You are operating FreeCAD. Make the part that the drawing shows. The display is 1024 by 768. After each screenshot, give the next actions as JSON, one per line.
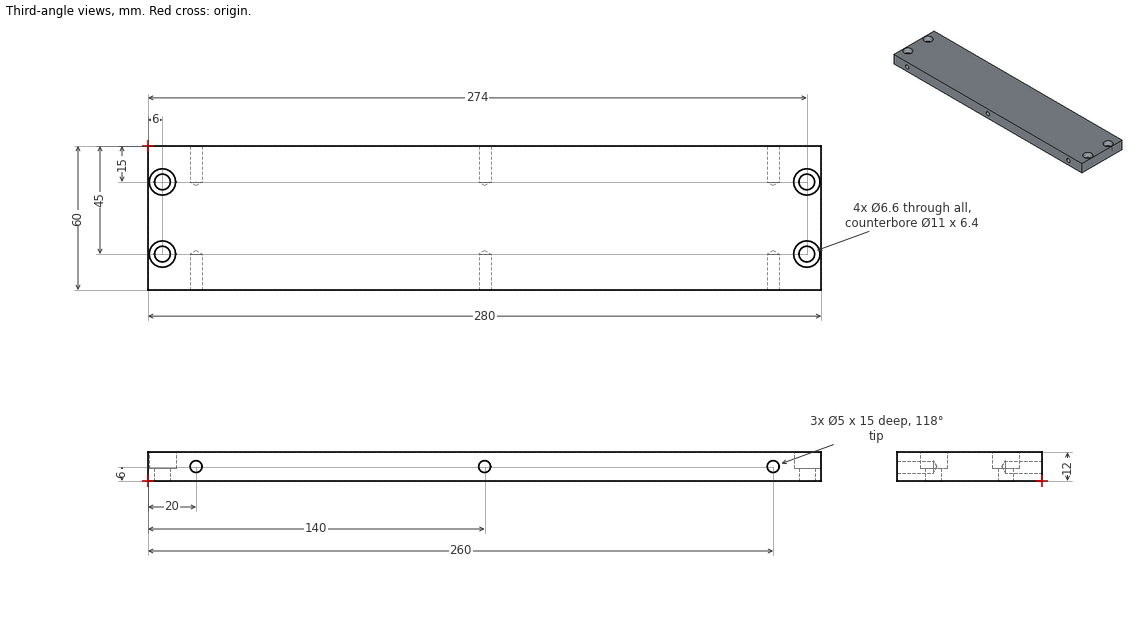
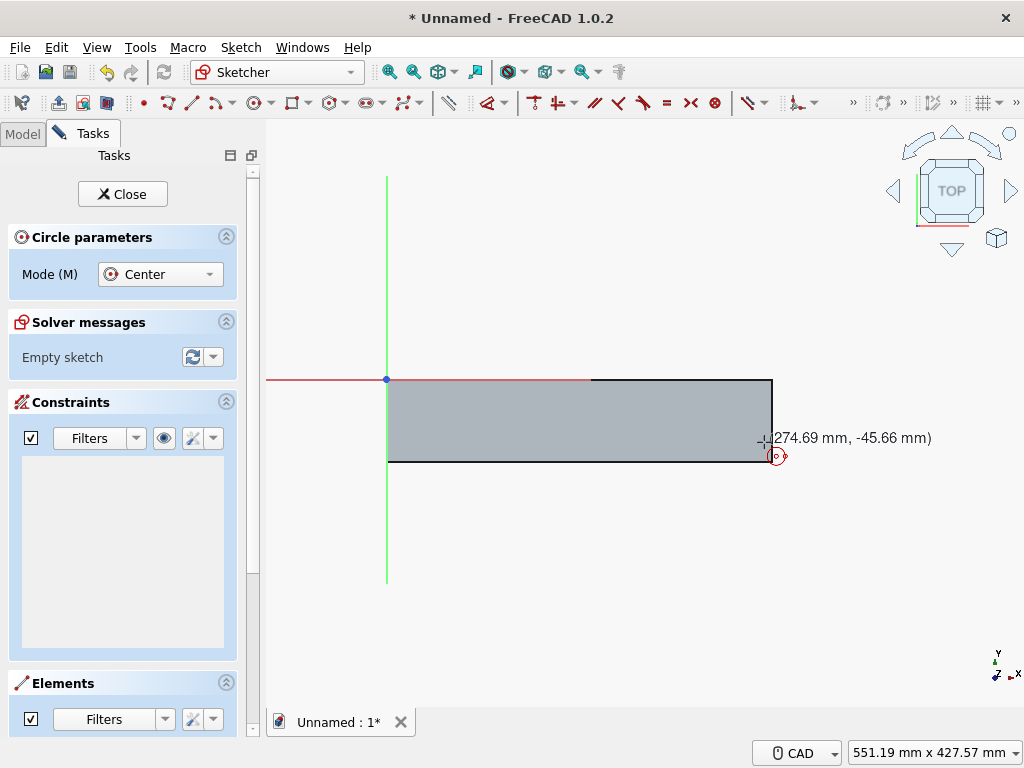
{"action": "left_click", "coordinate": [764, 442]}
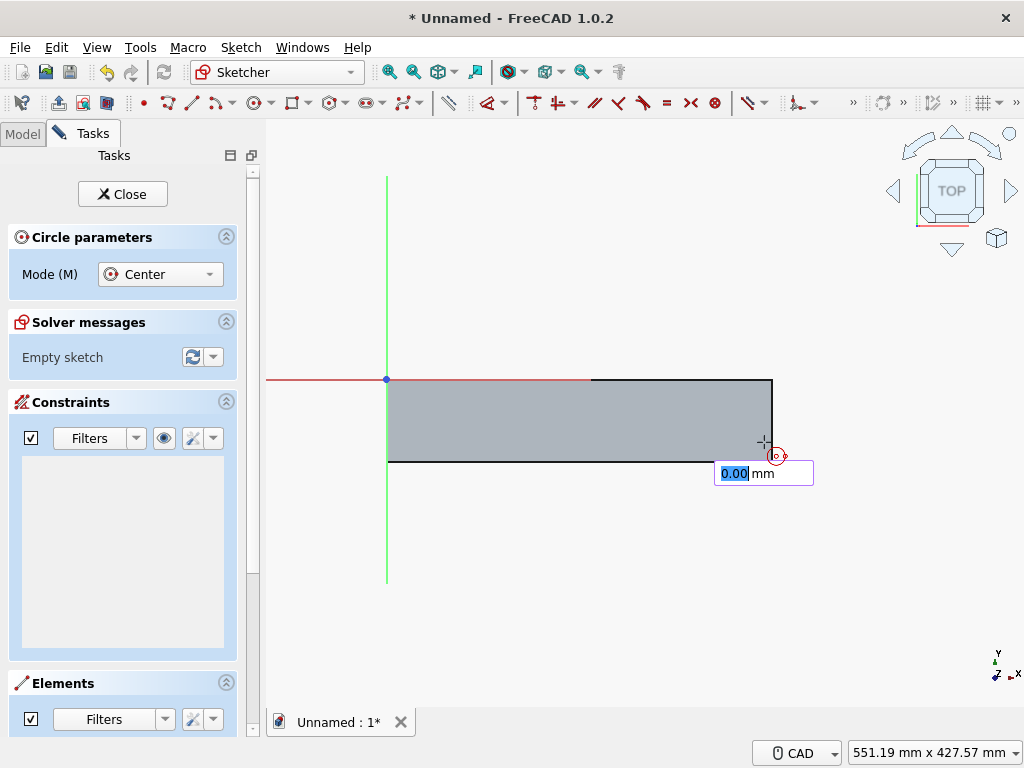
{"action": "scroll", "coordinate": [767, 439], "scroll_direction": "up", "scroll_amount": 7}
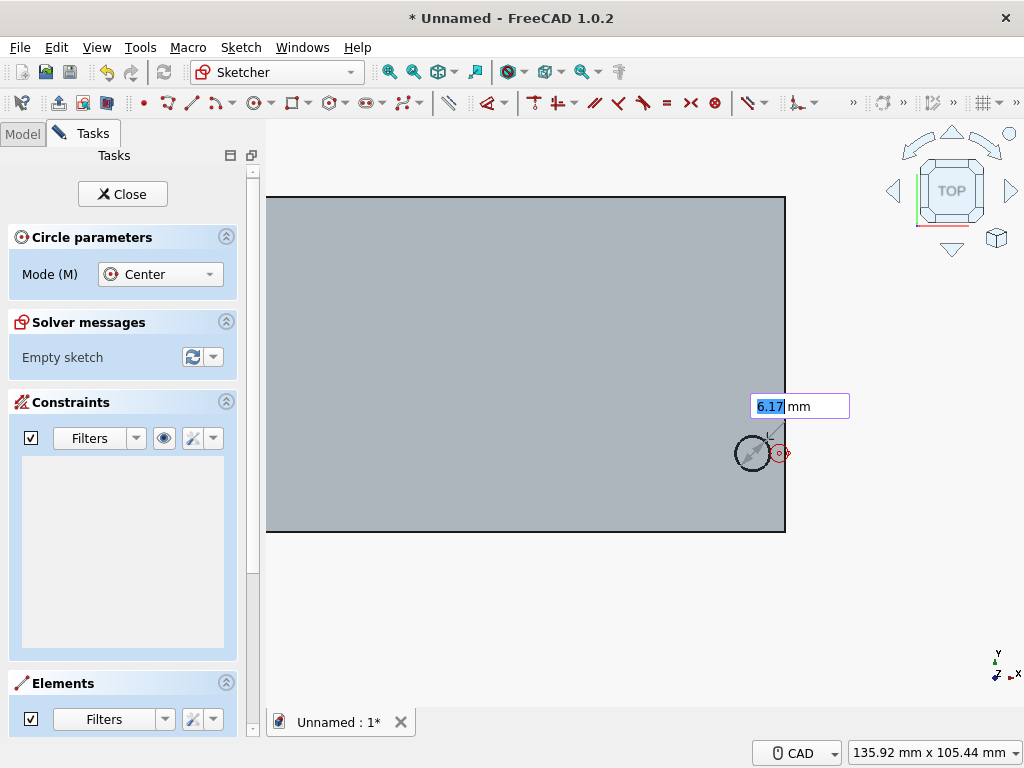
{"action": "left_click", "coordinate": [764, 435]}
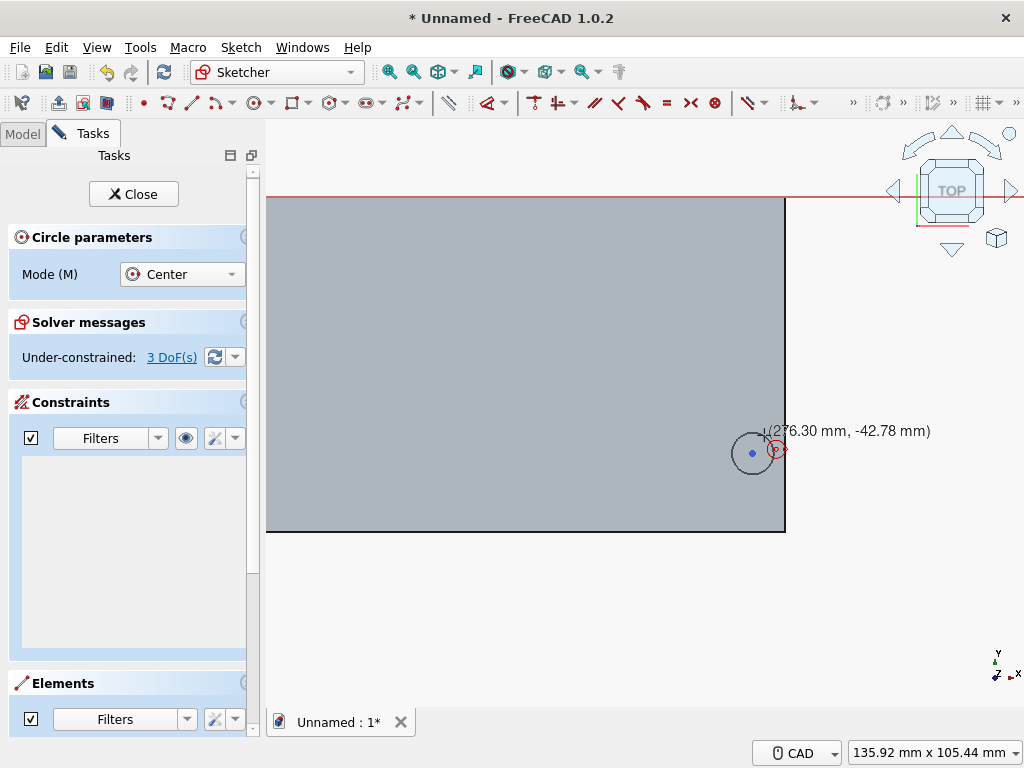
{"action": "scroll", "coordinate": [751, 281], "scroll_direction": "up", "scroll_amount": 2}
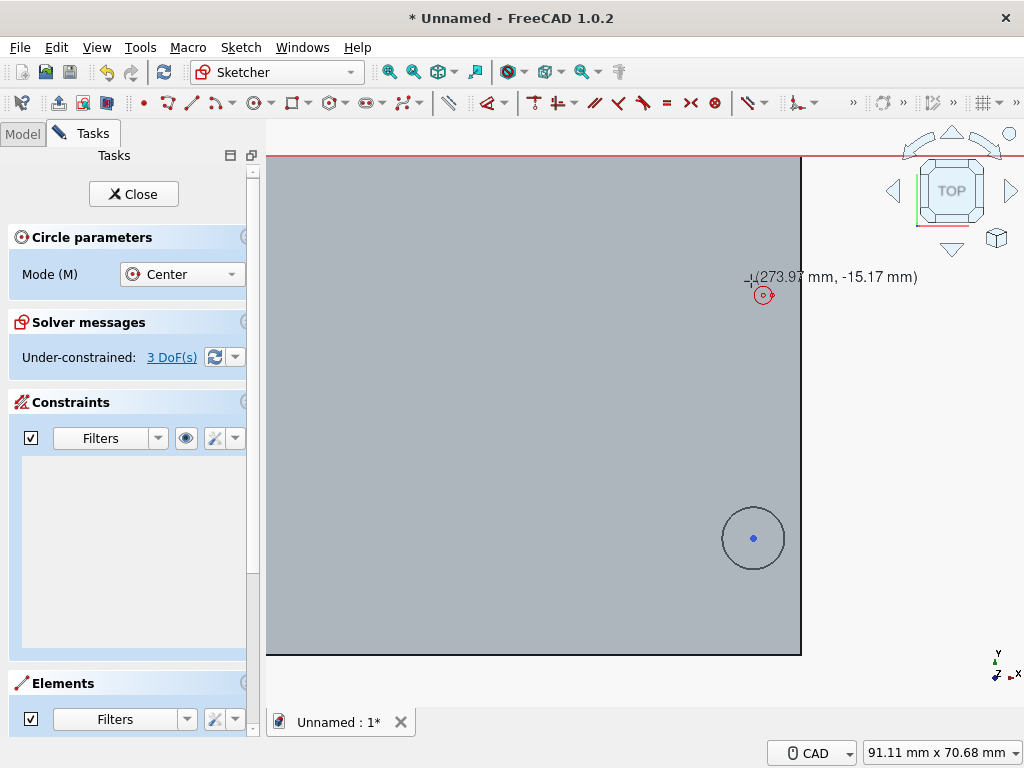
{"action": "scroll", "coordinate": [765, 424], "scroll_direction": "down", "scroll_amount": 9}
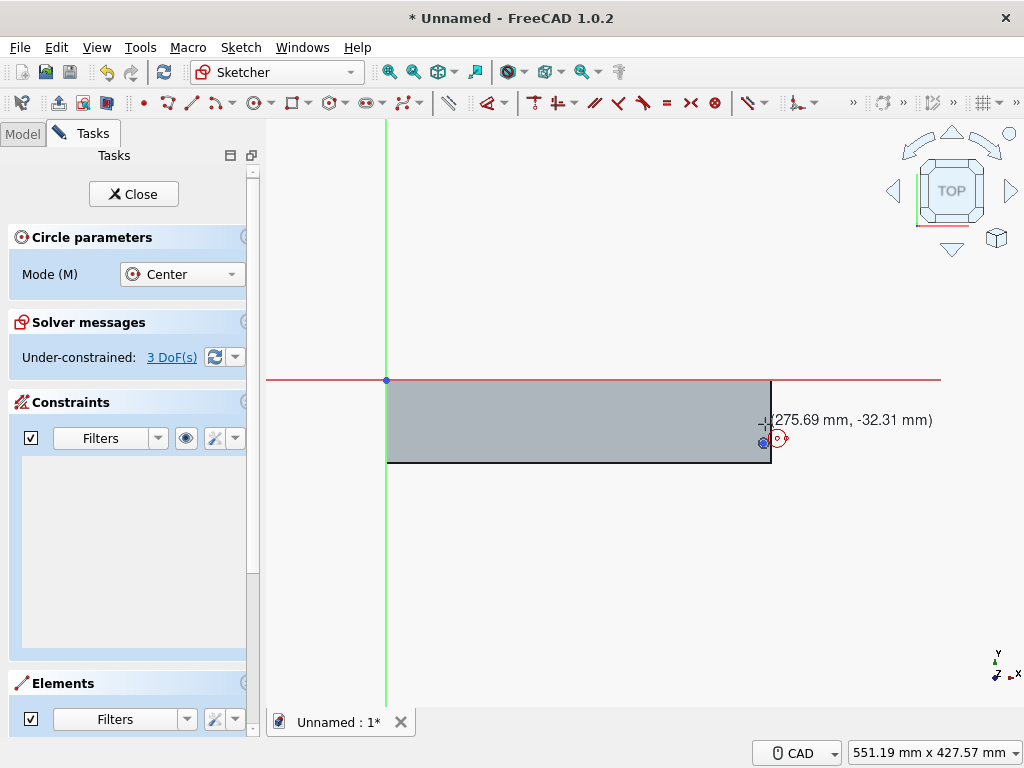
{"action": "left_click", "coordinate": [763, 401]}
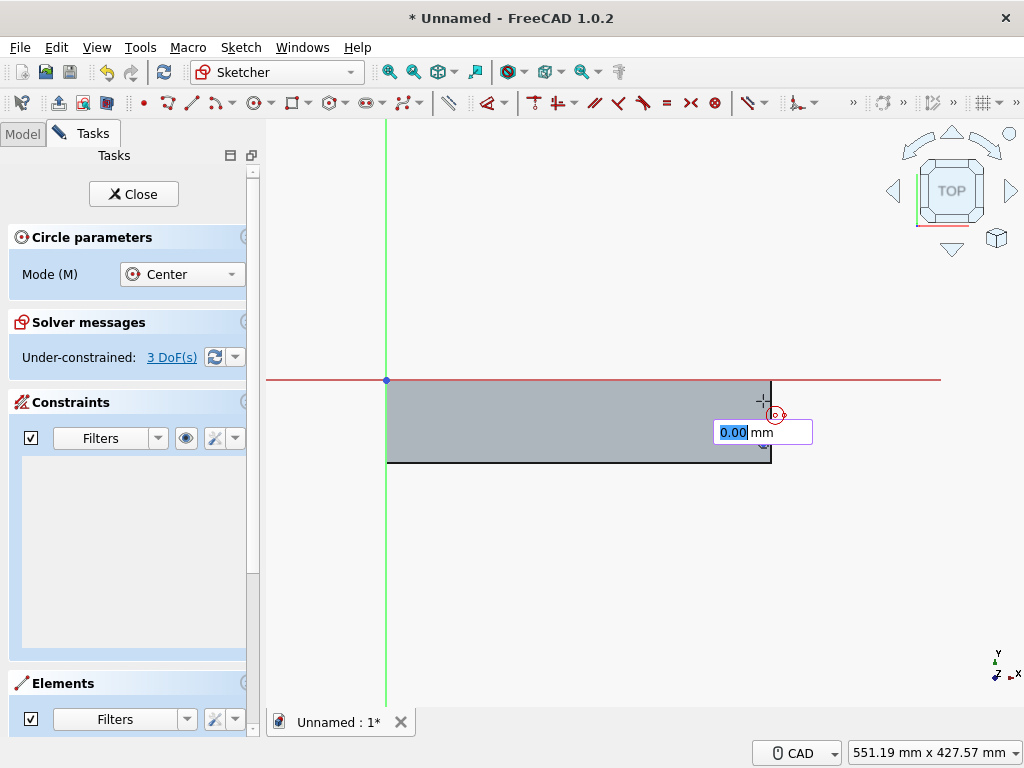
{"action": "scroll", "coordinate": [766, 398], "scroll_direction": "up", "scroll_amount": 7}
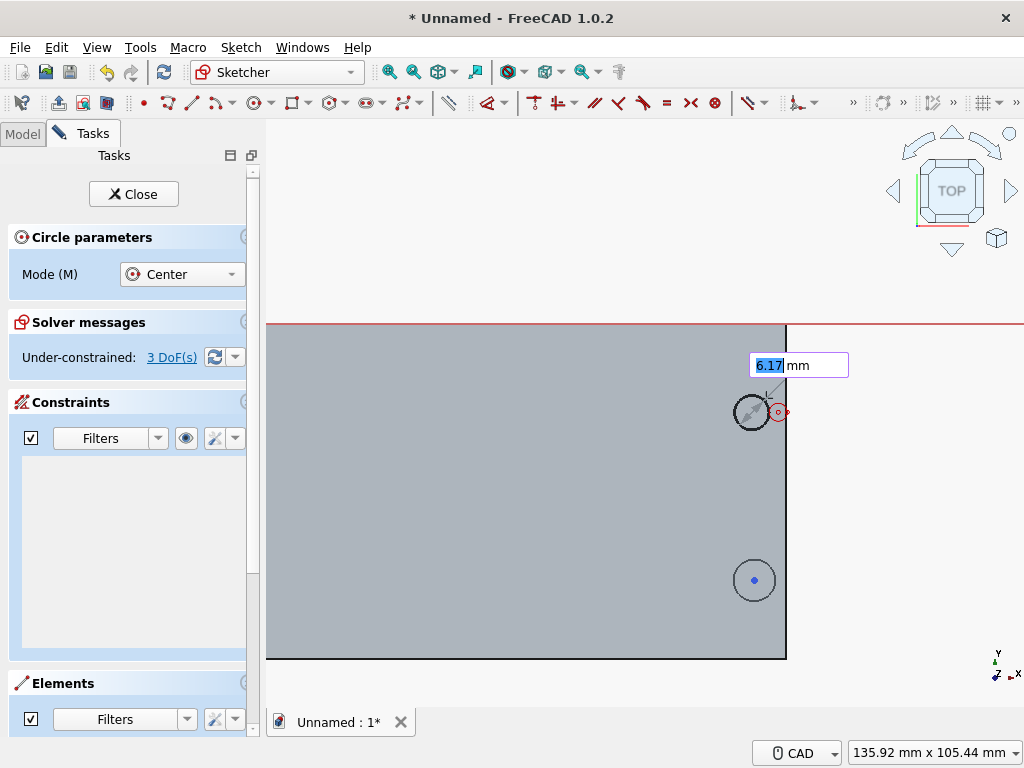
{"action": "left_click", "coordinate": [766, 395]}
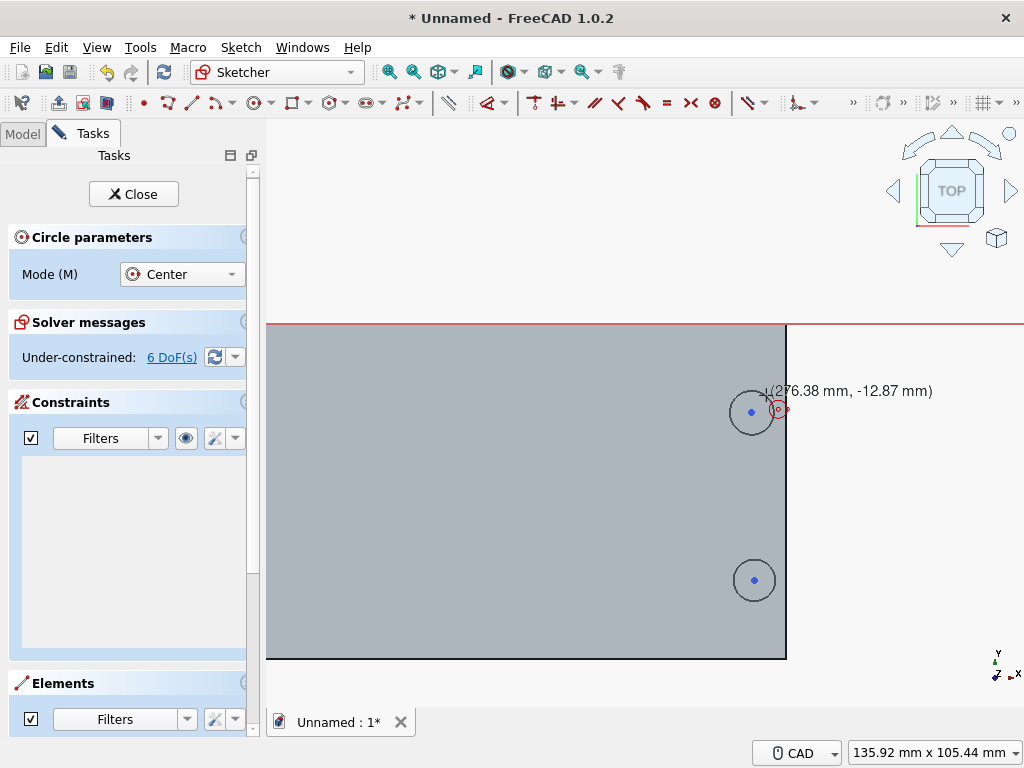
{"action": "scroll", "coordinate": [766, 398], "scroll_direction": "down", "scroll_amount": 7}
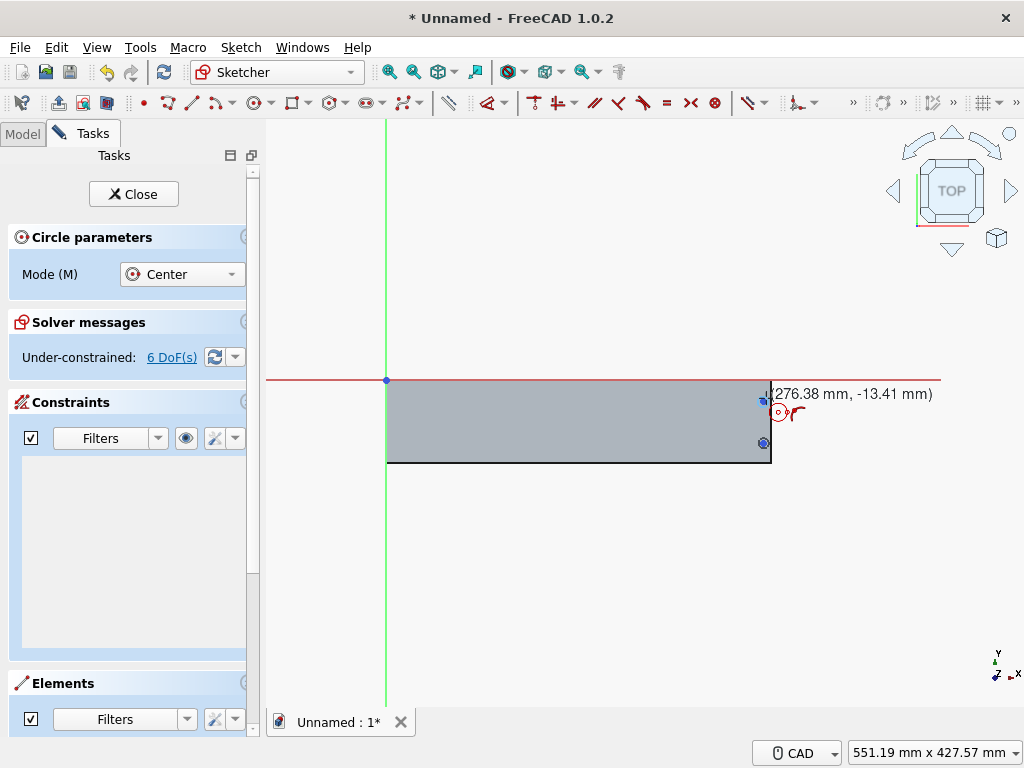
{"action": "scroll", "coordinate": [395, 442], "scroll_direction": "up", "scroll_amount": 9}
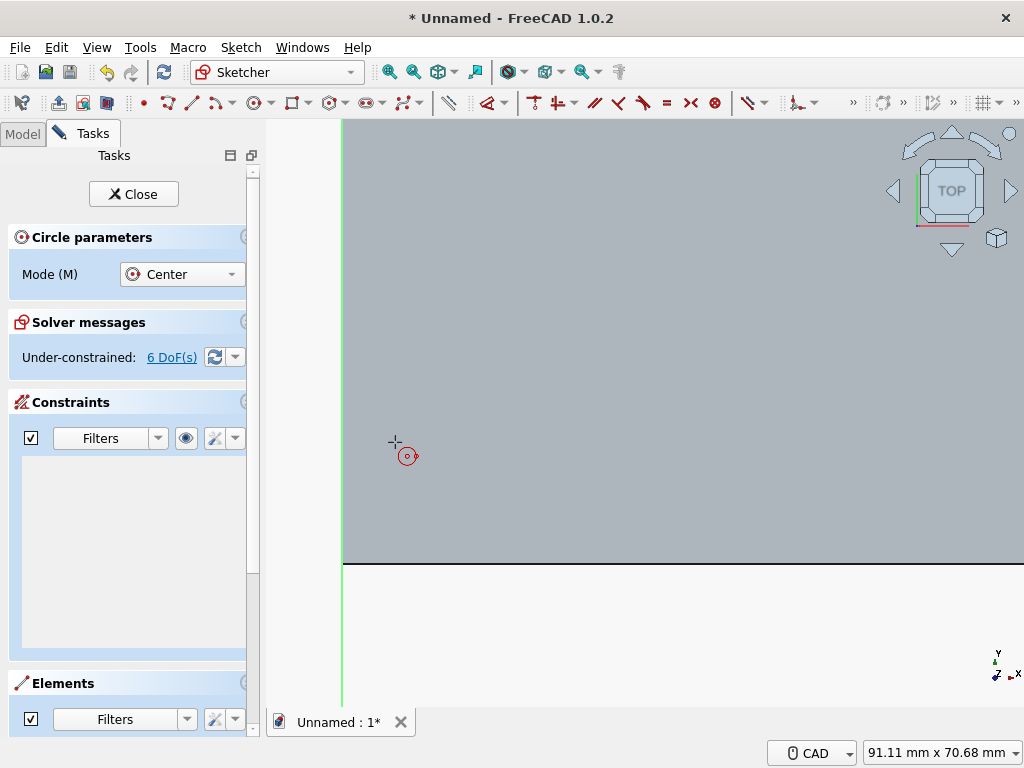
{"action": "scroll", "coordinate": [394, 442], "scroll_direction": "down", "scroll_amount": 9}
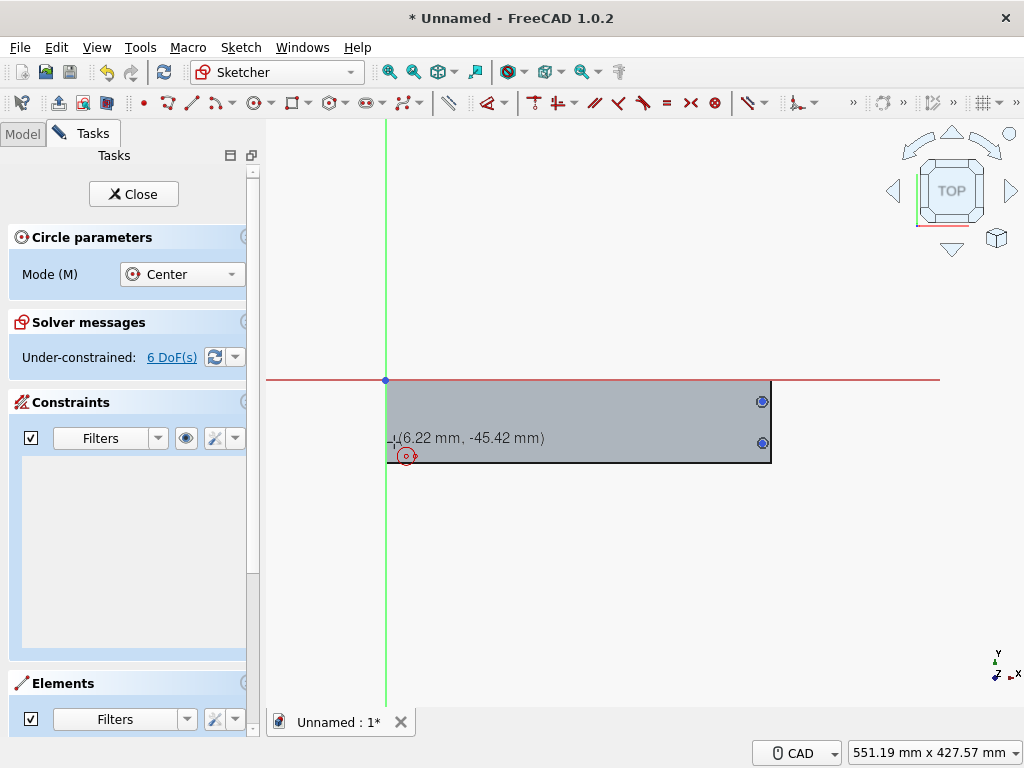
{"action": "scroll", "coordinate": [394, 442], "scroll_direction": "up", "scroll_amount": 4}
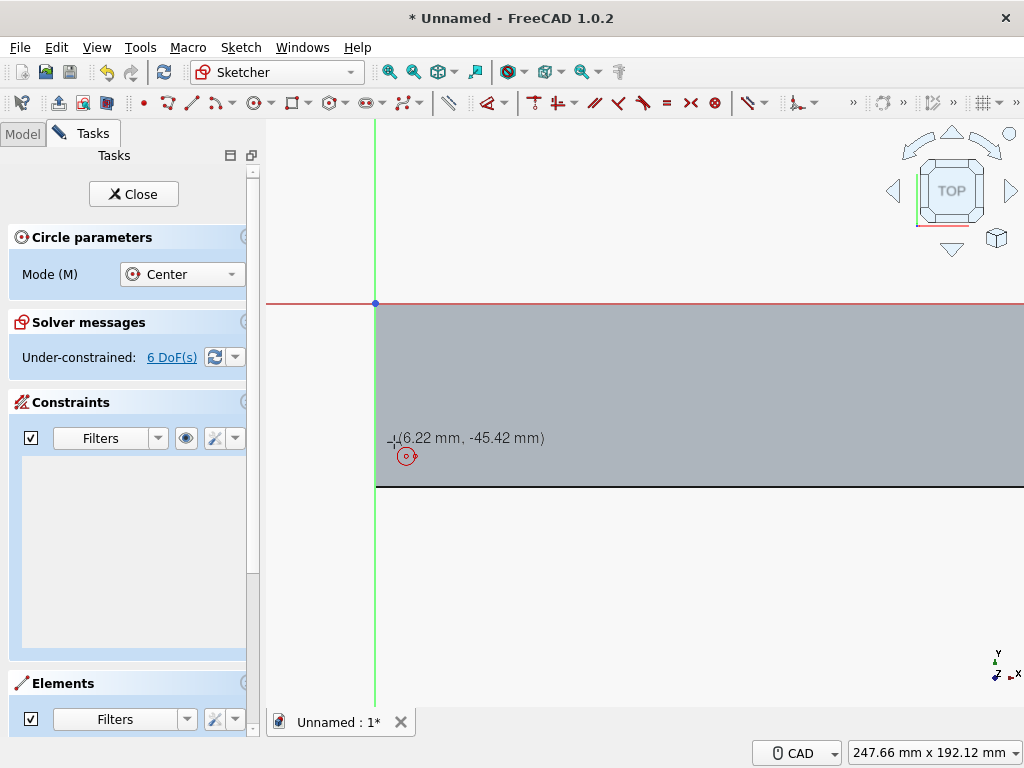
{"action": "left_click", "coordinate": [393, 441]}